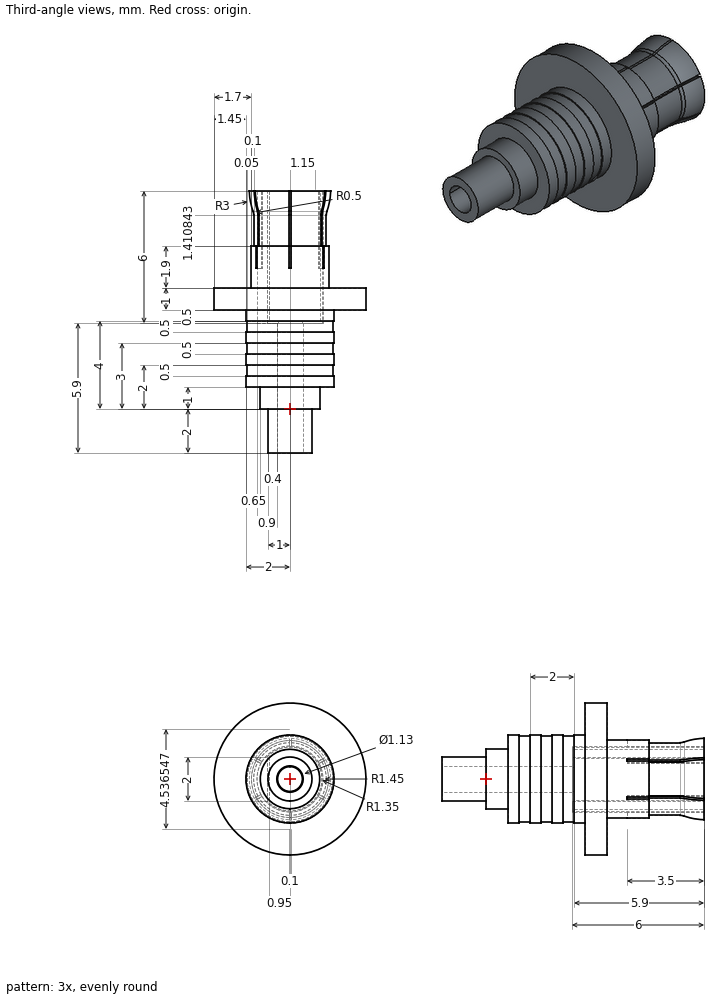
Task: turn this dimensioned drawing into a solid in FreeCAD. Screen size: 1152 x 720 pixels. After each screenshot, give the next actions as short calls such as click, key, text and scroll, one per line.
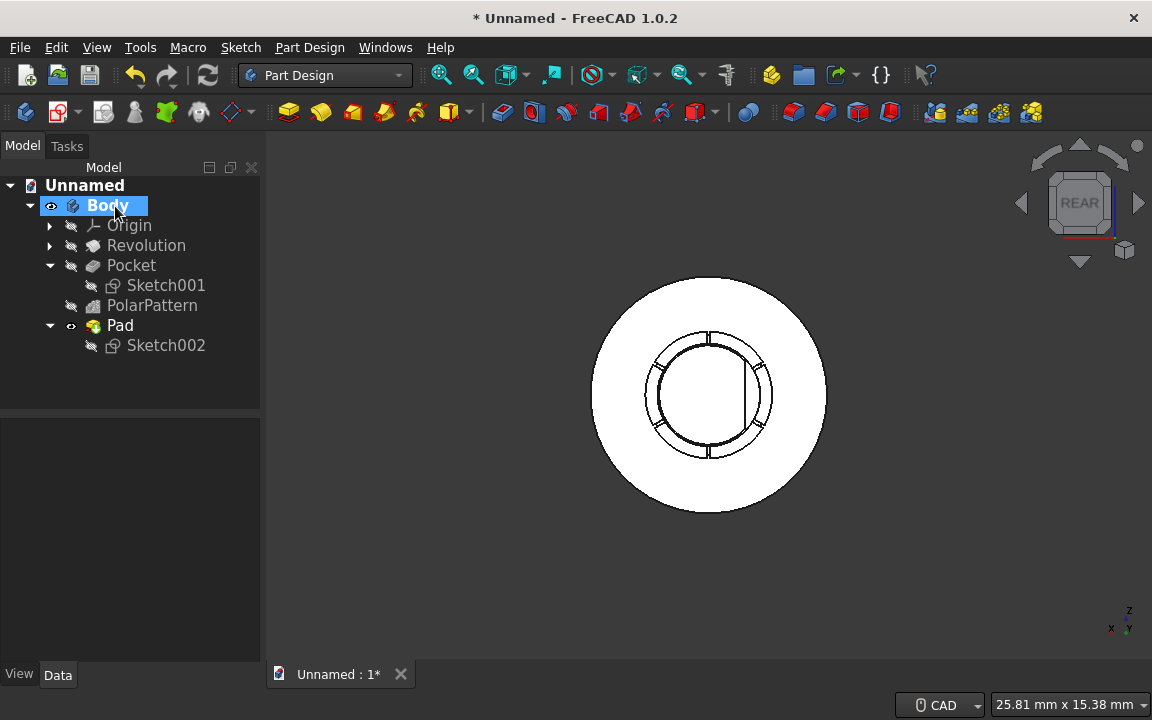
click(442, 76)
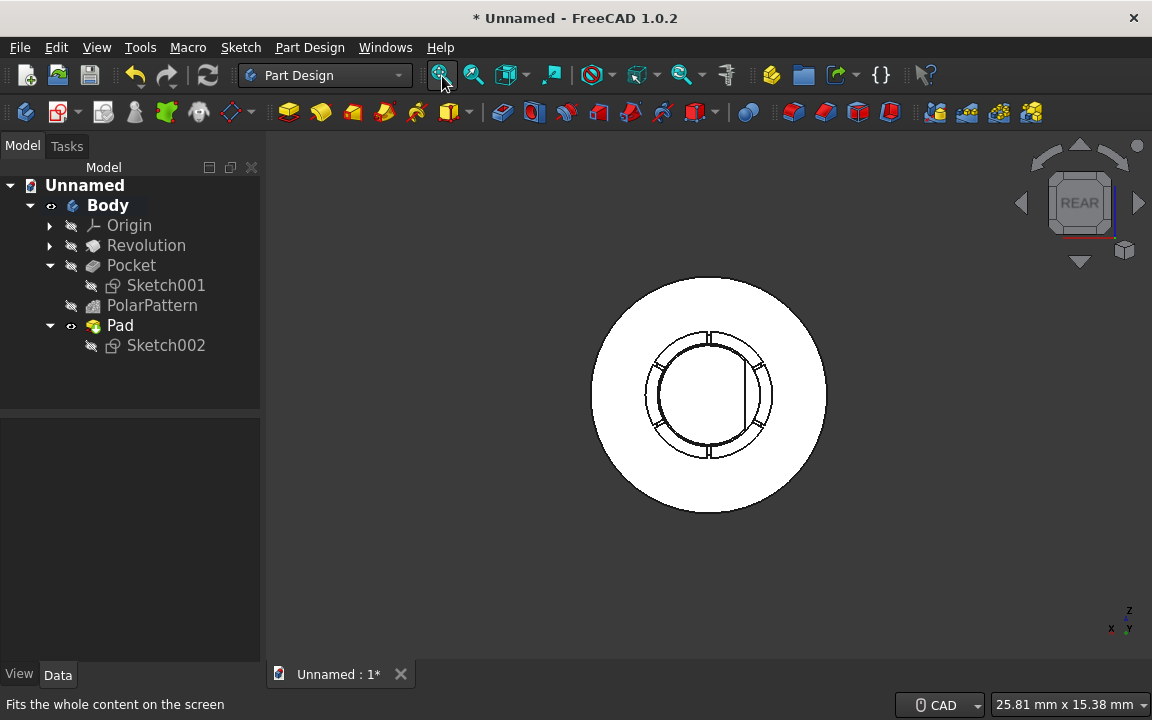
click(702, 394)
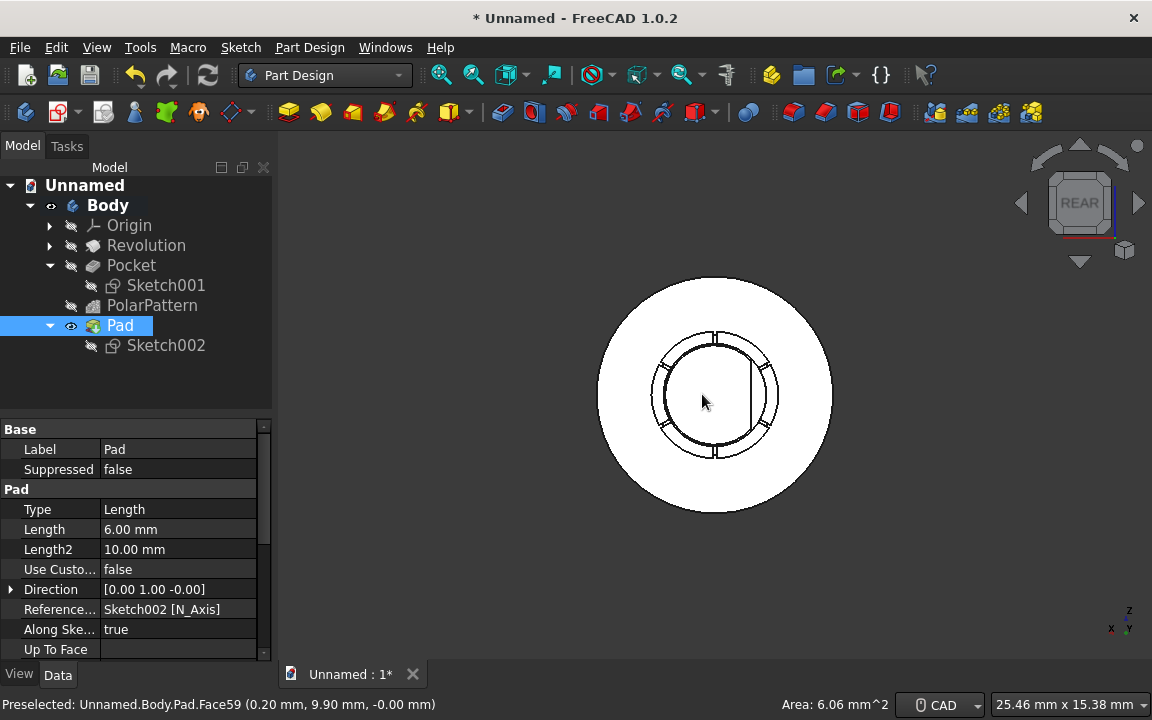
click(58, 112)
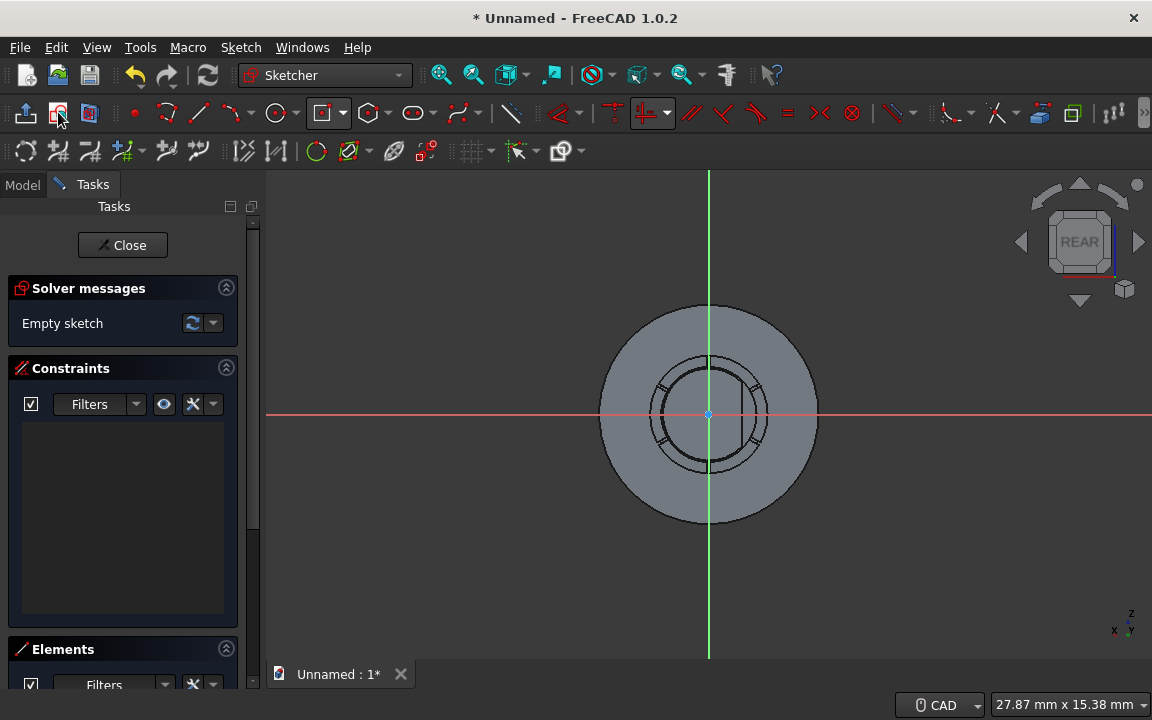
scroll(718, 415, up, 8)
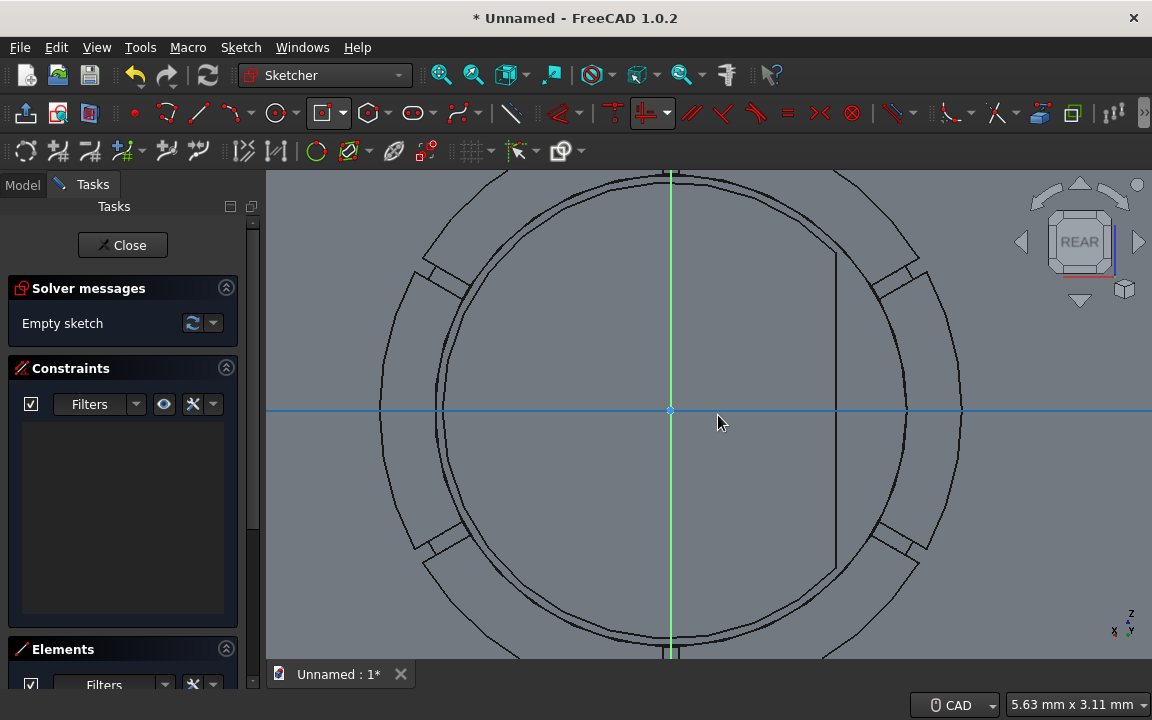
click(200, 114)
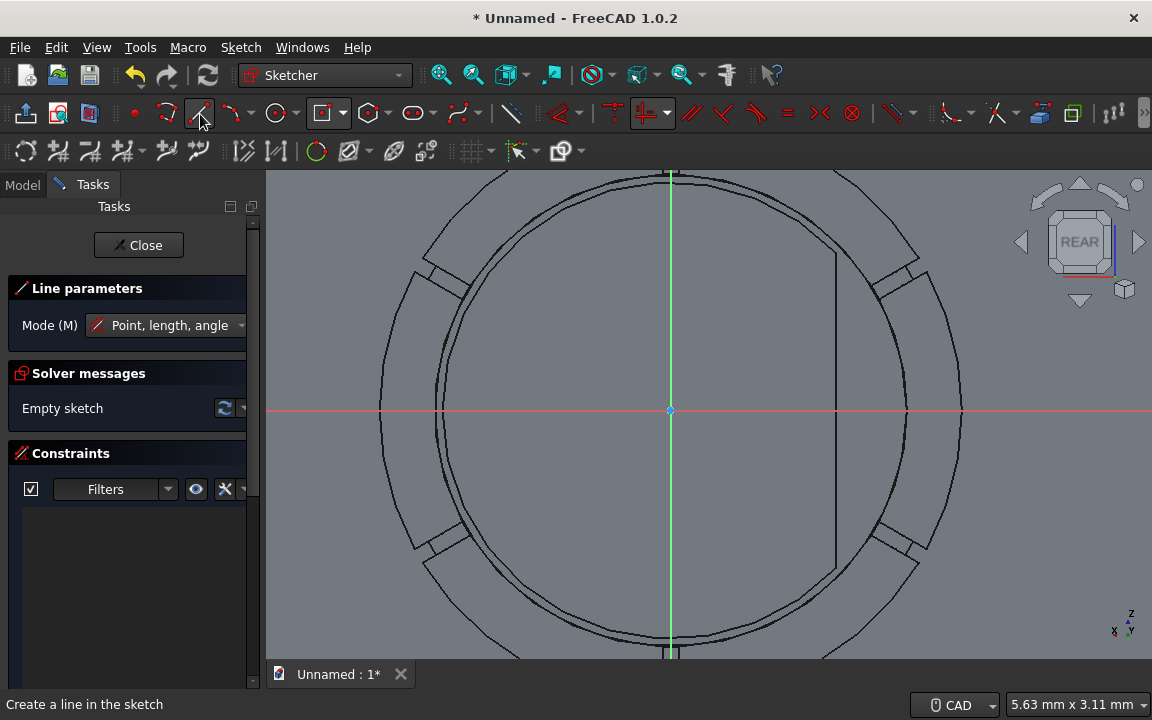
click(820, 562)
click(820, 260)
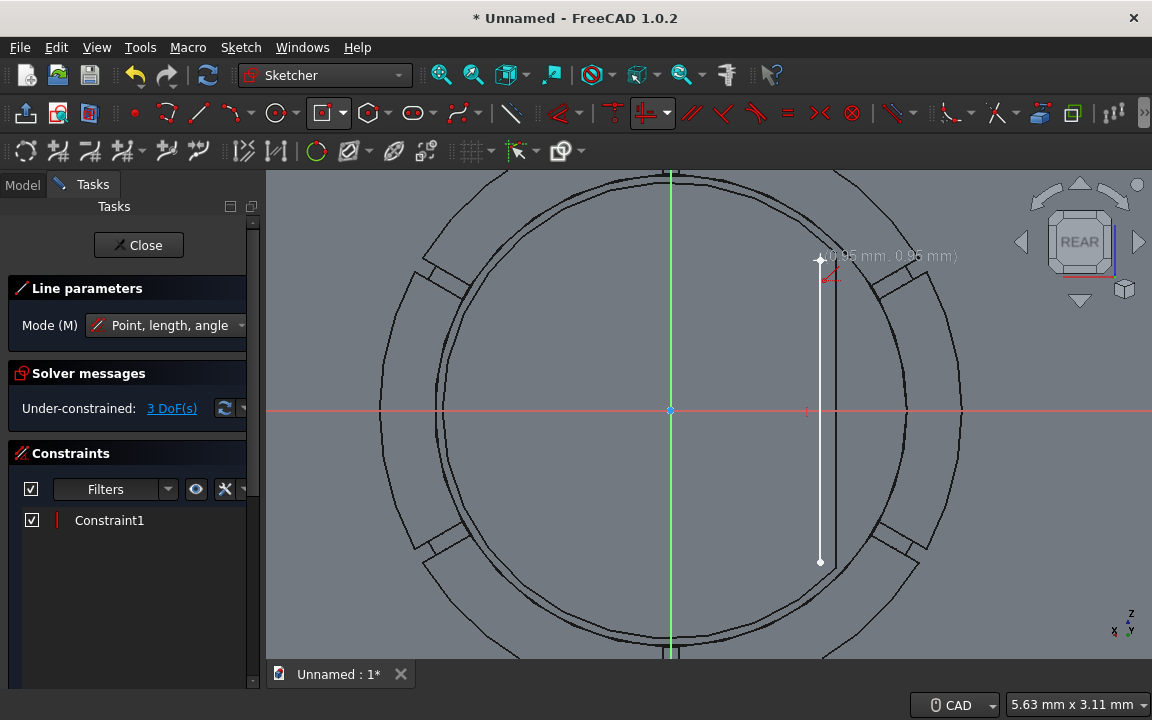
click(232, 114)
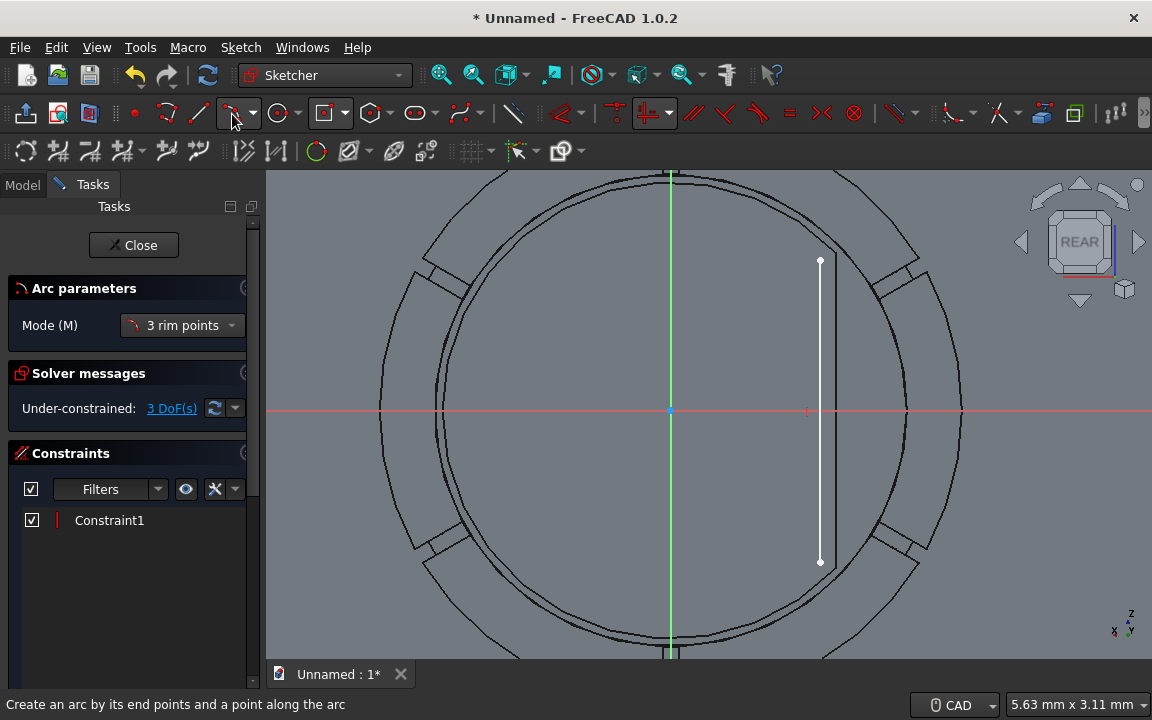
click(820, 261)
click(820, 563)
click(481, 314)
key(Escape)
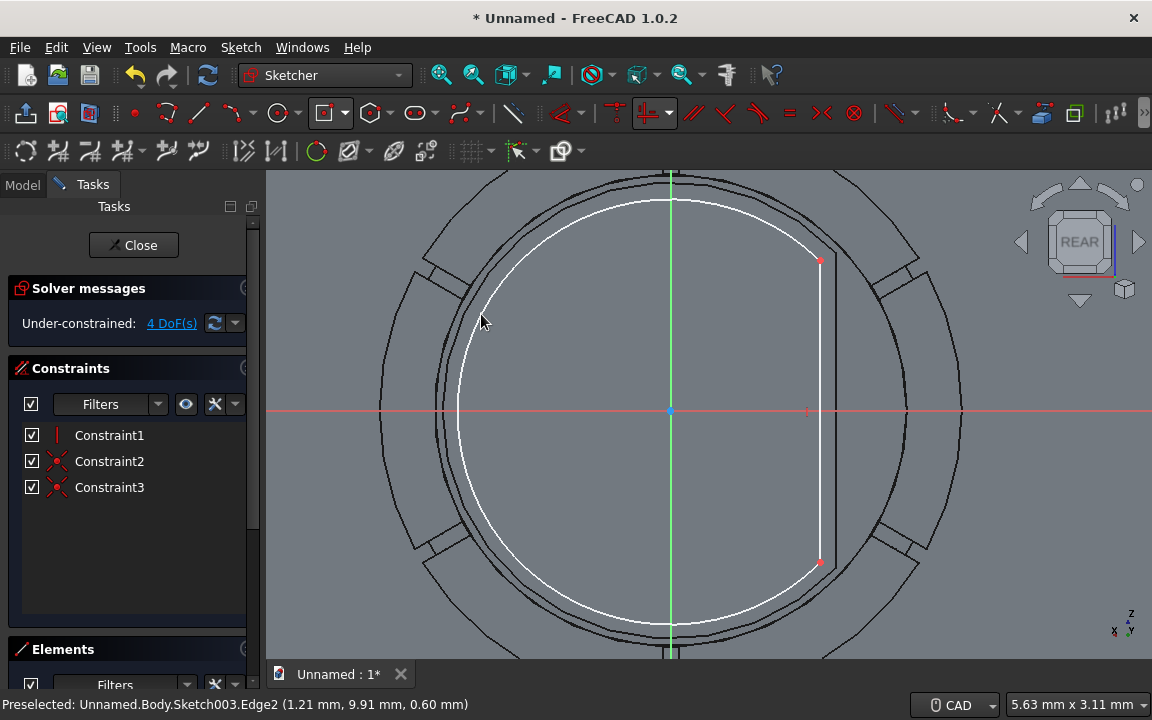
drag(660, 401, 681, 422)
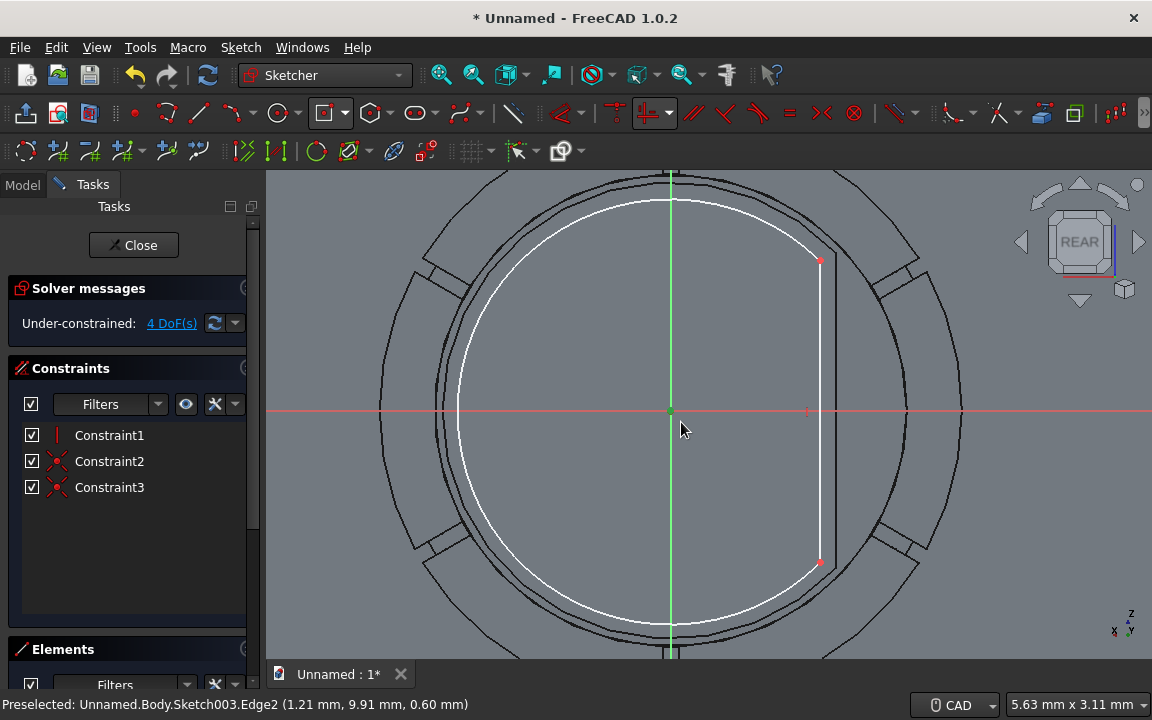
click(616, 114)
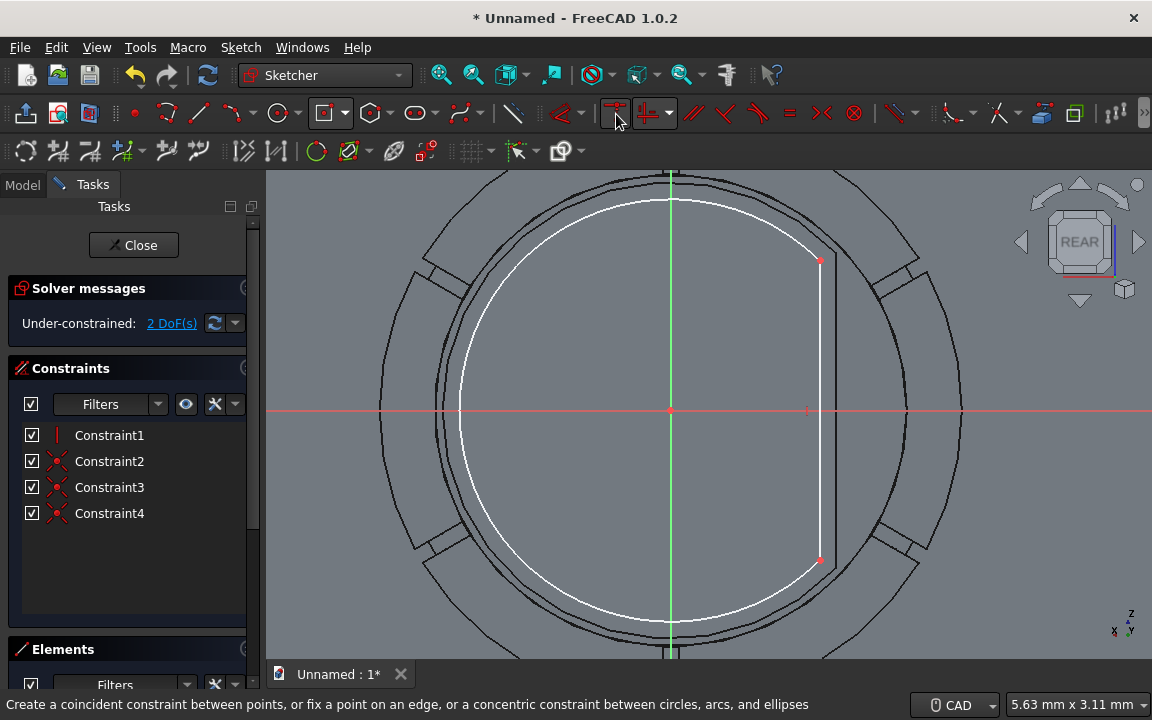
click(560, 114)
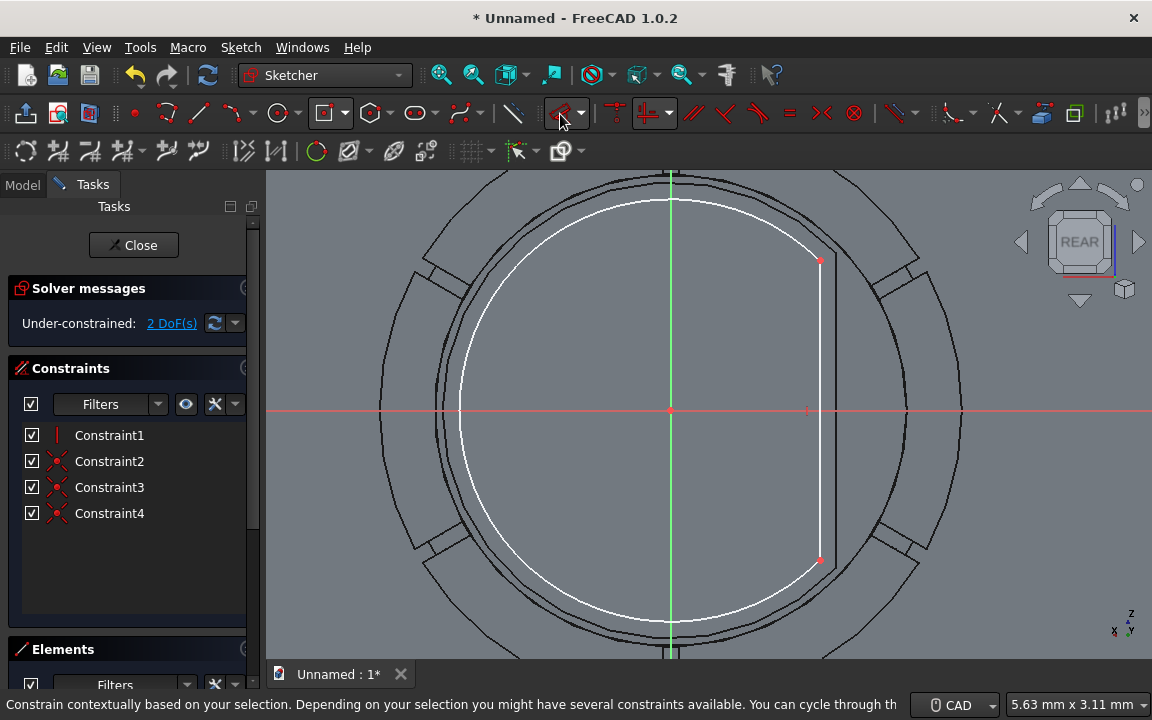
click(546, 240)
click(527, 214)